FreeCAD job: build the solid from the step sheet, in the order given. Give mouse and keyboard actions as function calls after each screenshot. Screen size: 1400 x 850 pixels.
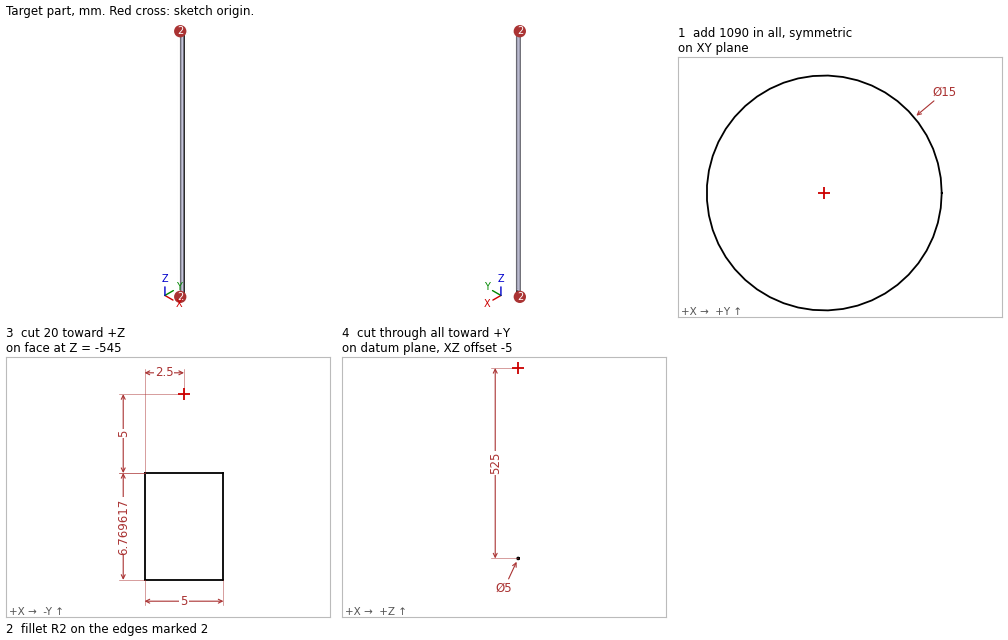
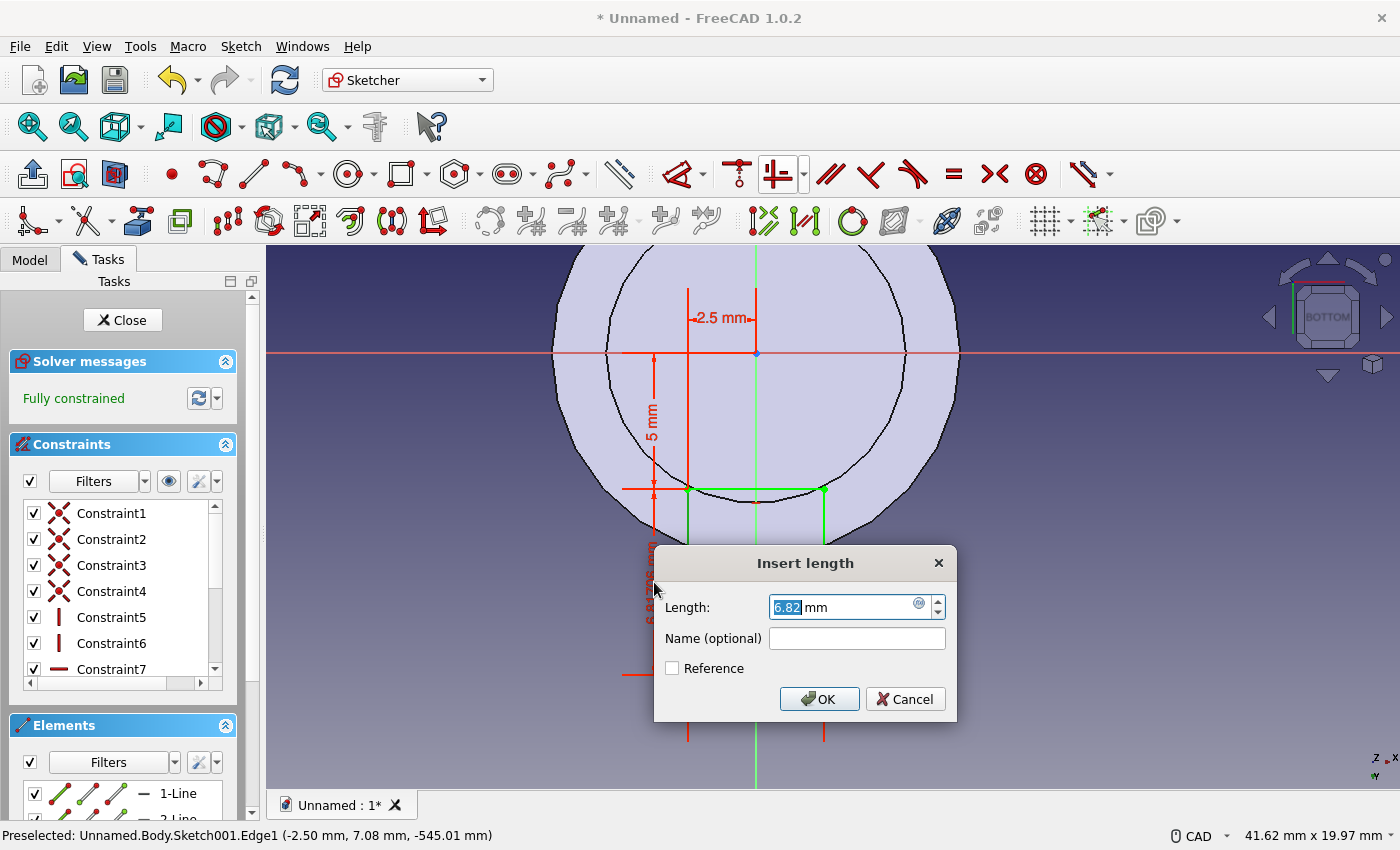
text(6.769617)
key(Return)
key(Escape)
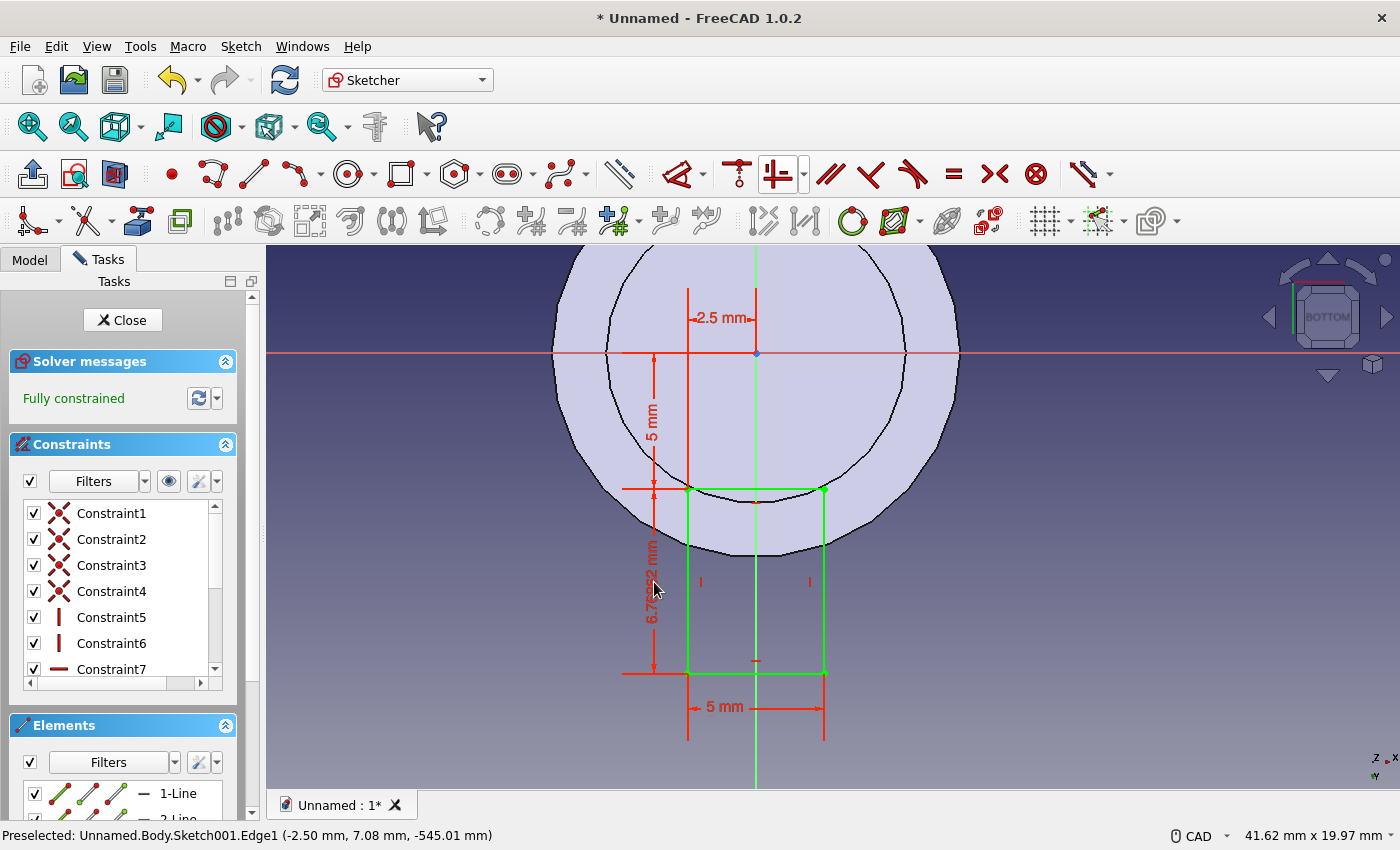
click(123, 320)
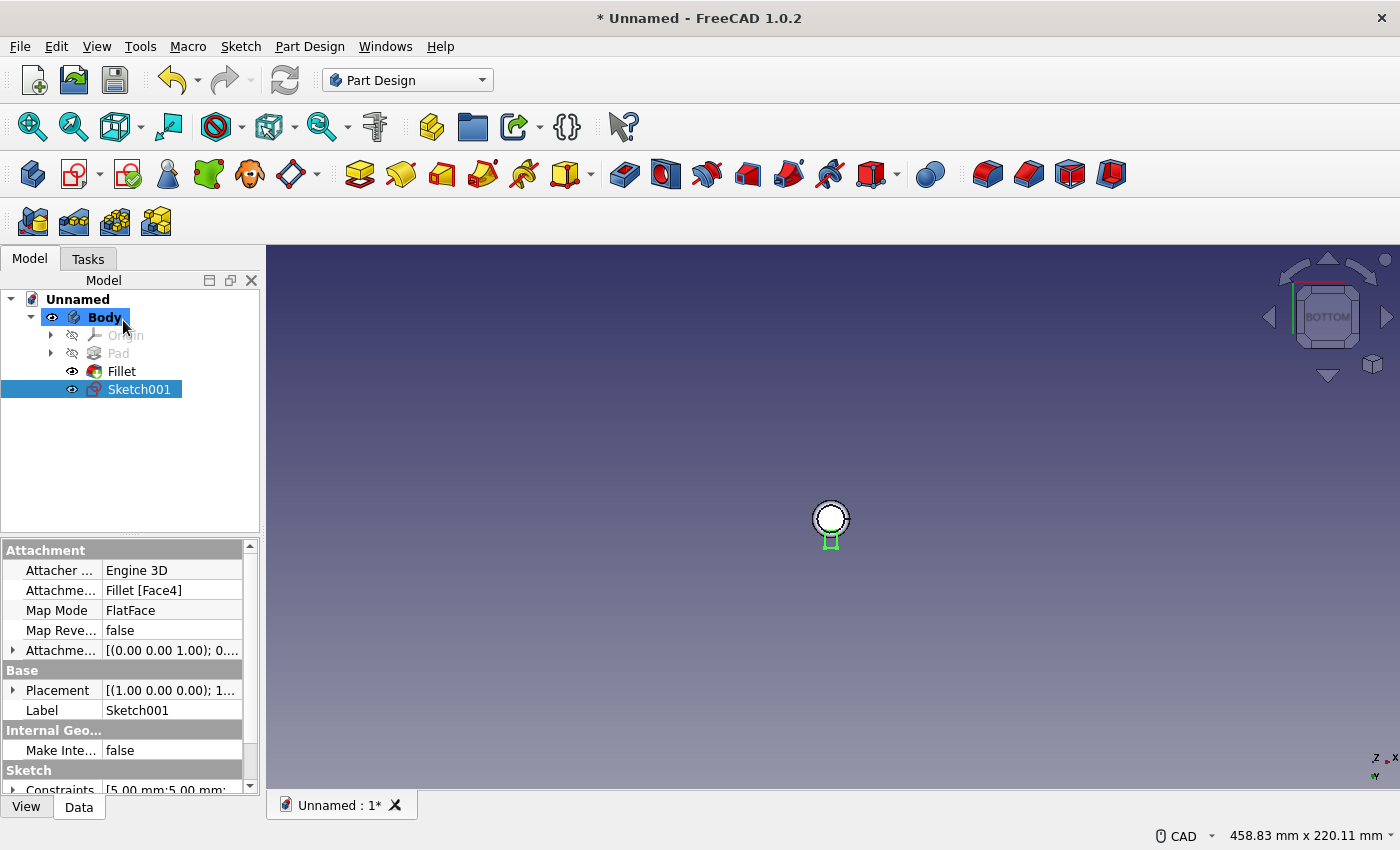
click(625, 174)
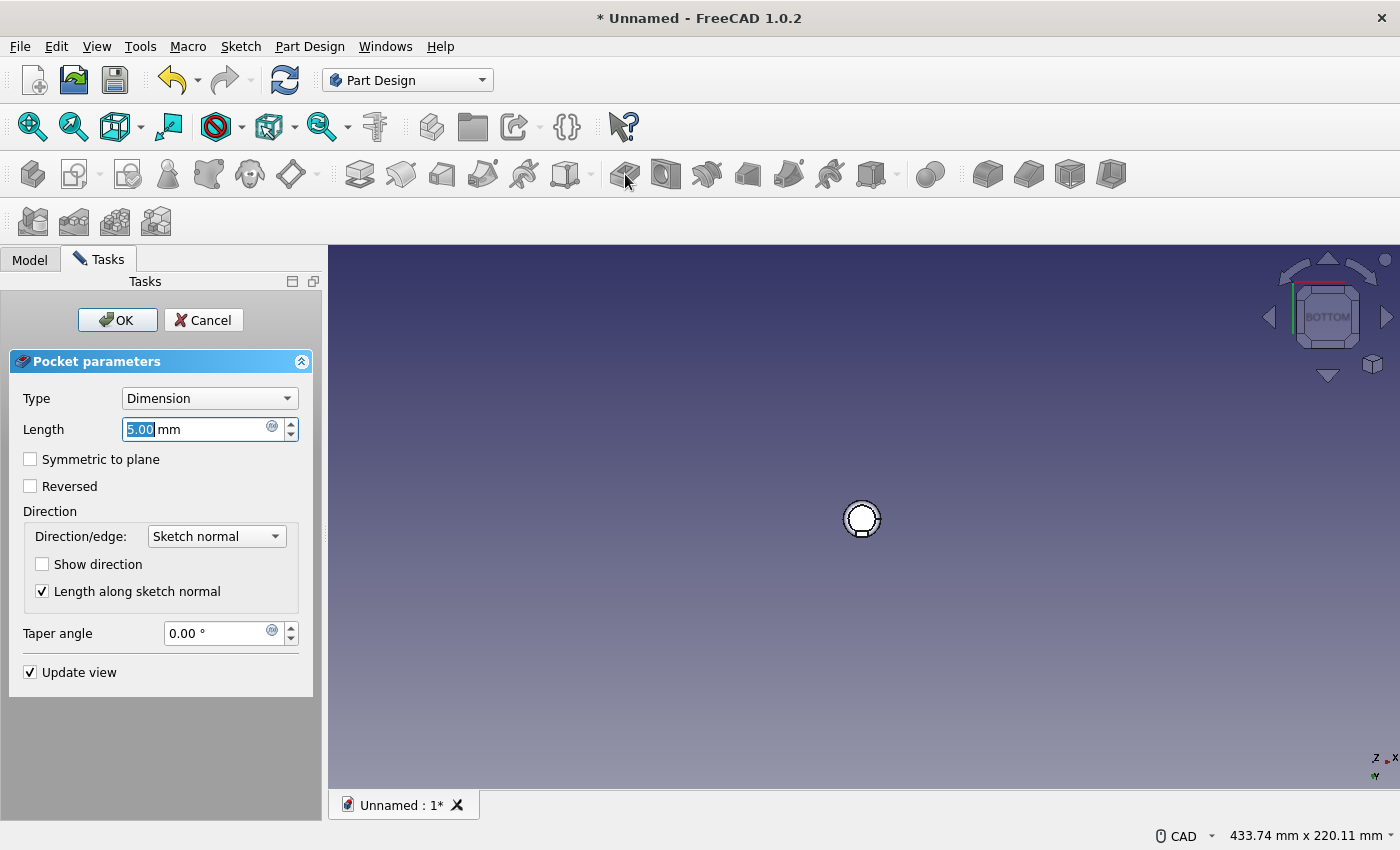
text(20)
key(Tab)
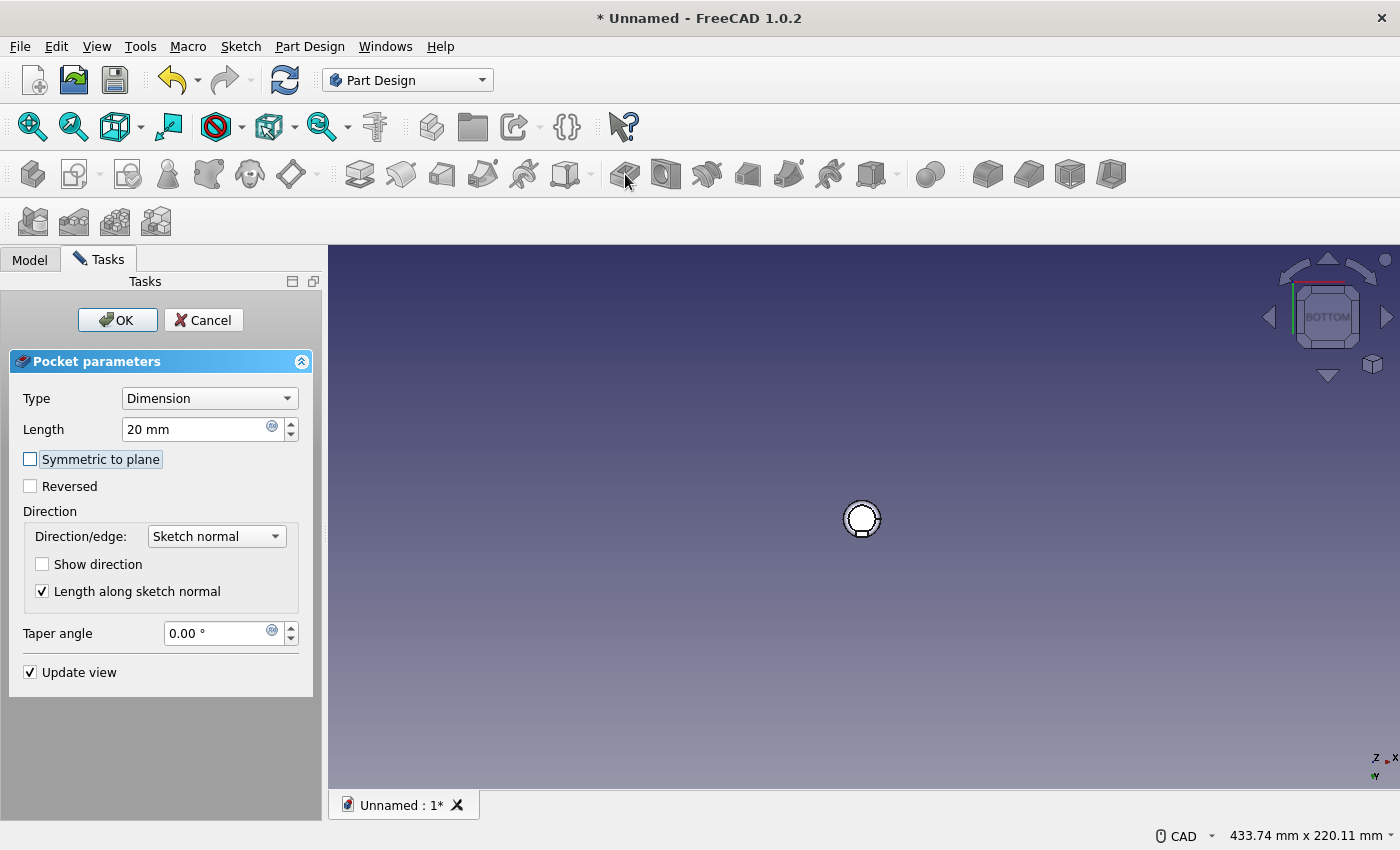
click(118, 320)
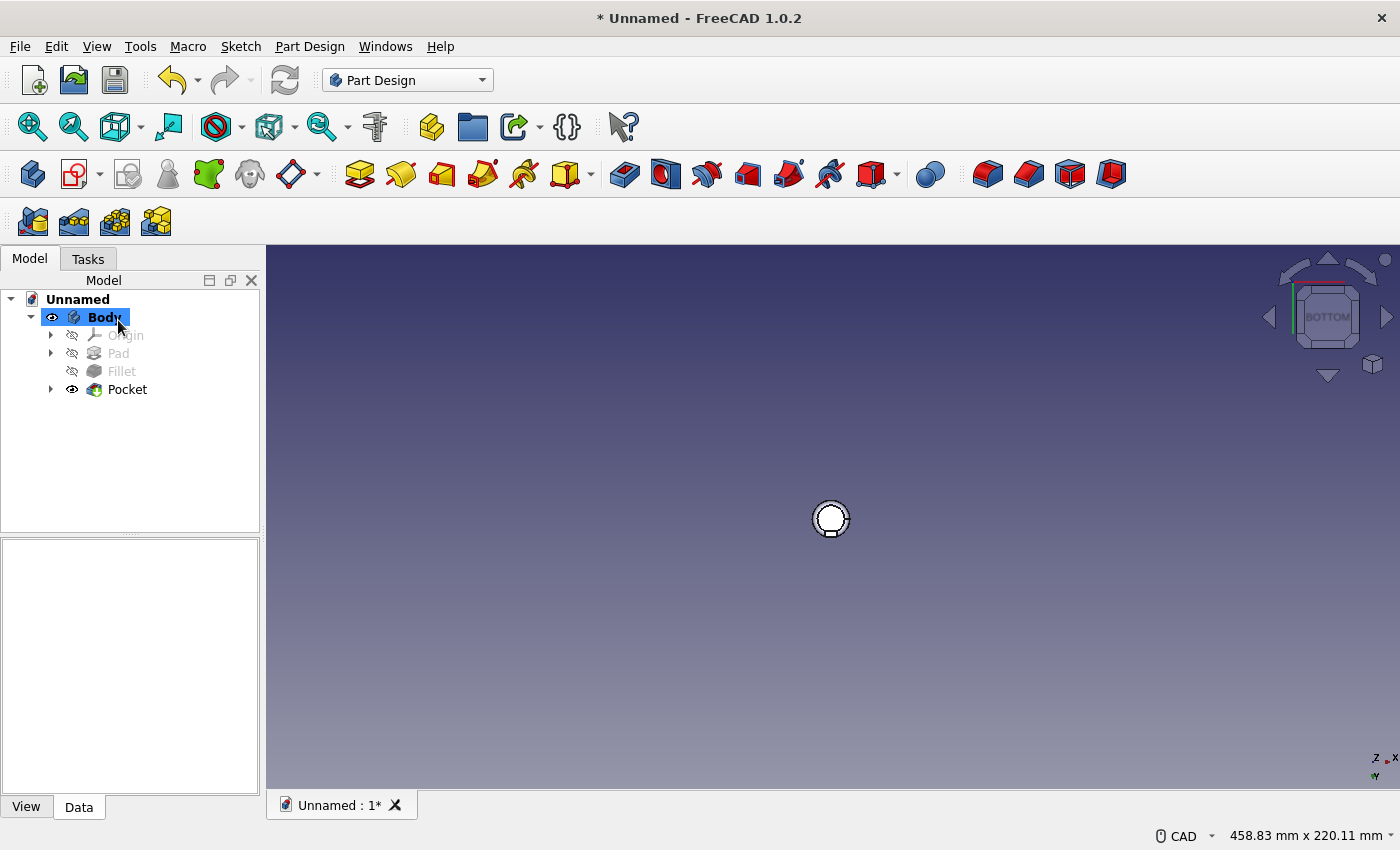
key(v)
key(f)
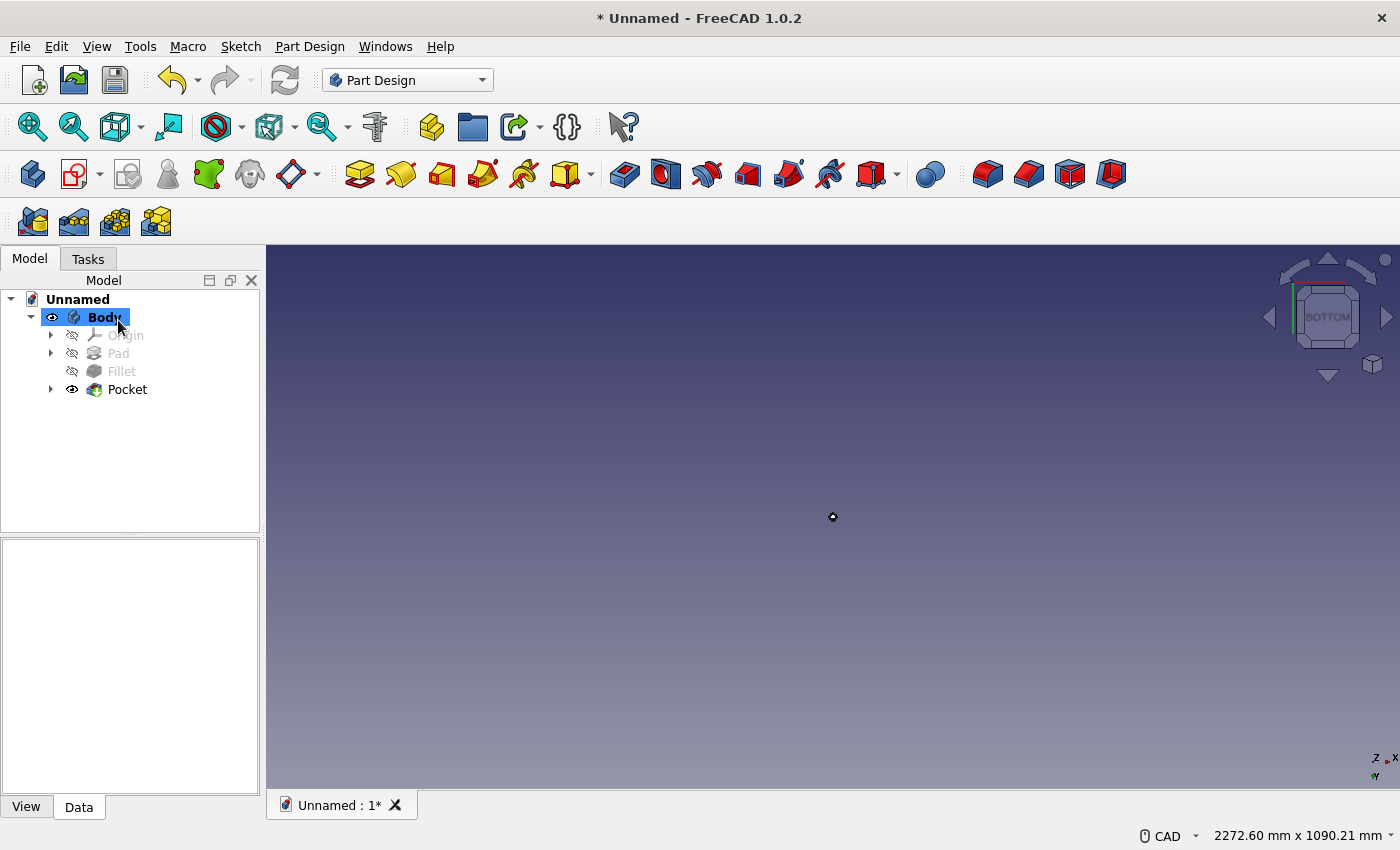
key(4)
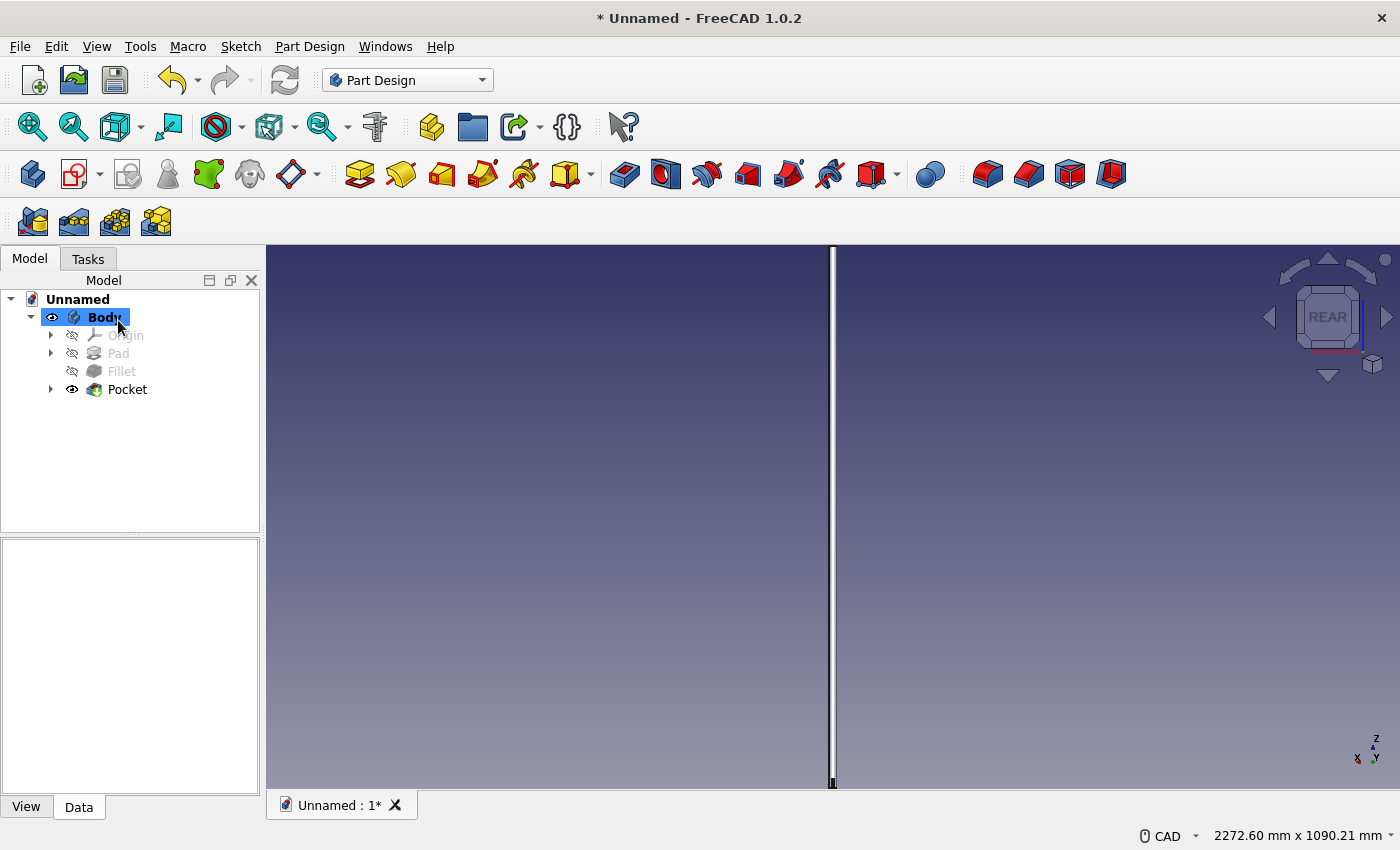
key(v)
key(f)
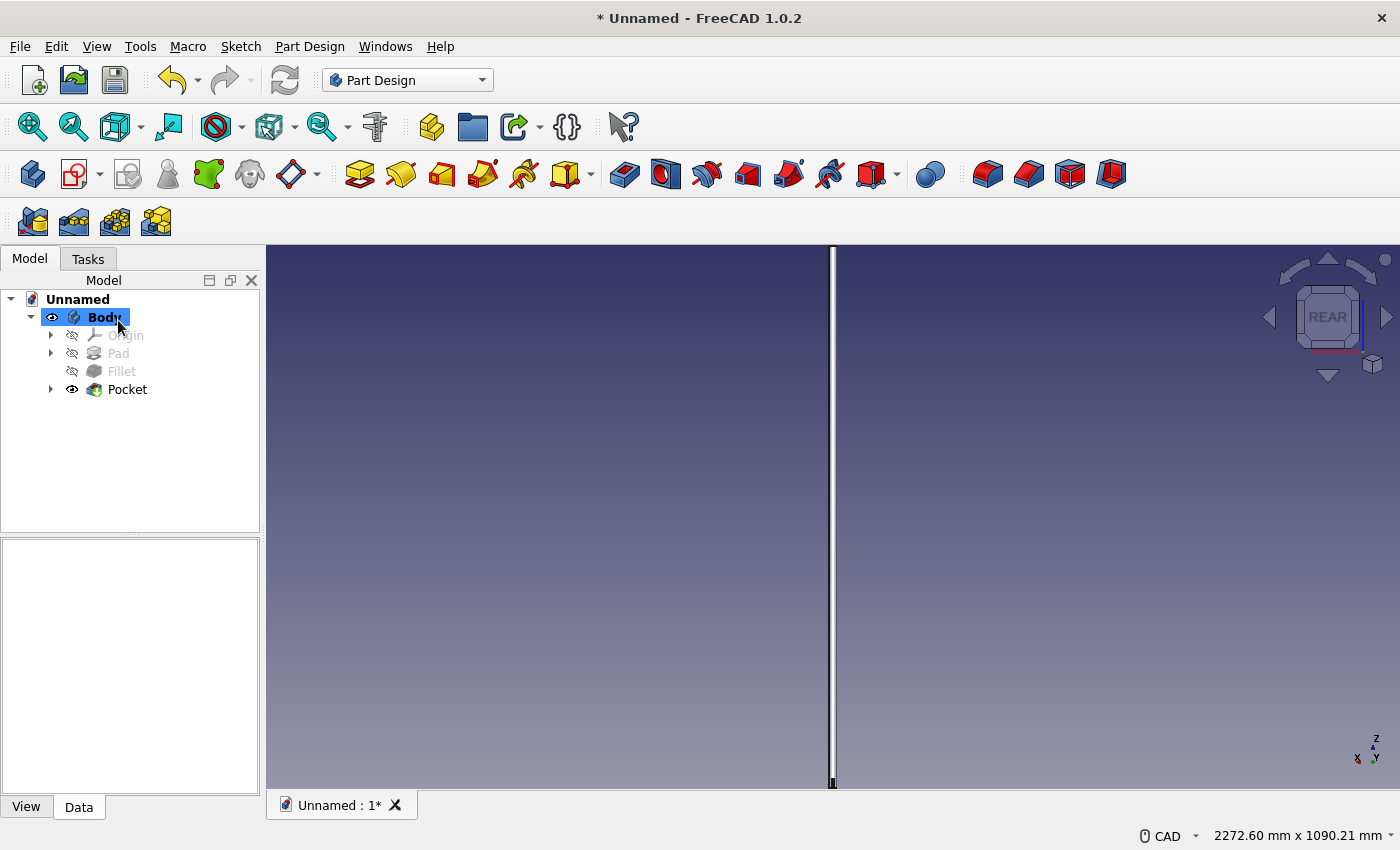
key(2)